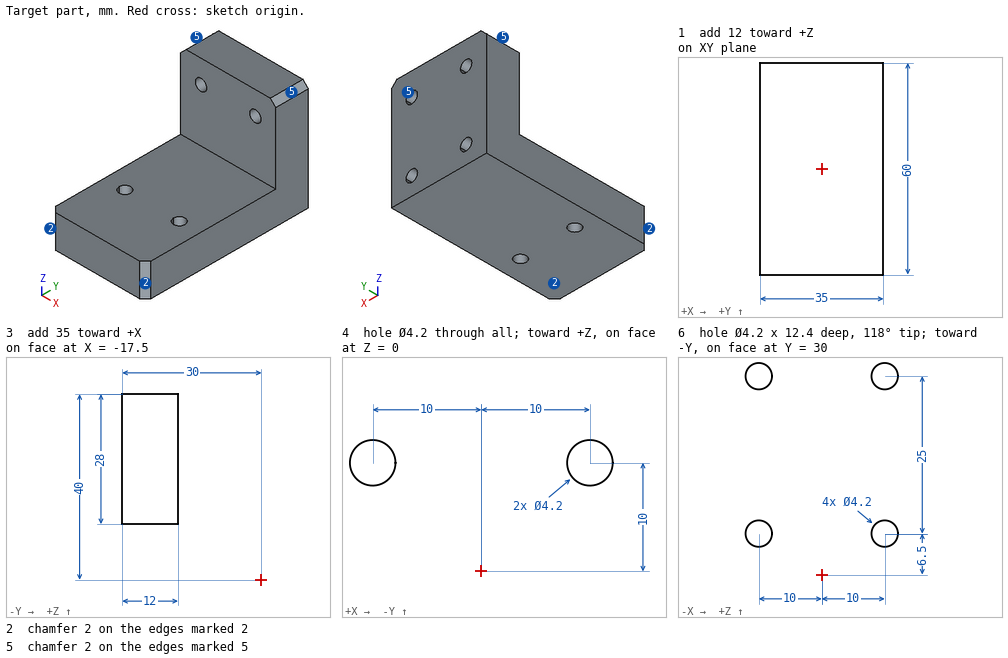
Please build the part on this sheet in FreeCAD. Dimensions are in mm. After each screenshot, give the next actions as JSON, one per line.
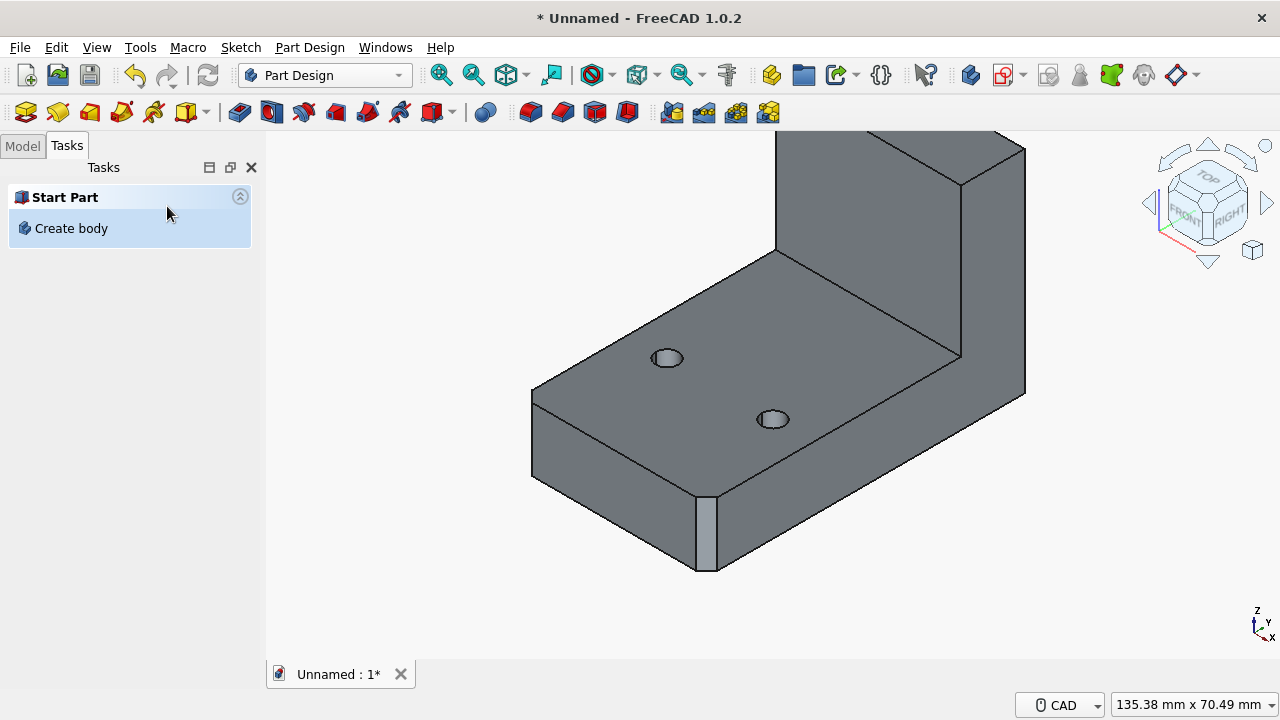
{"action": "left_click", "coordinate": [442, 76]}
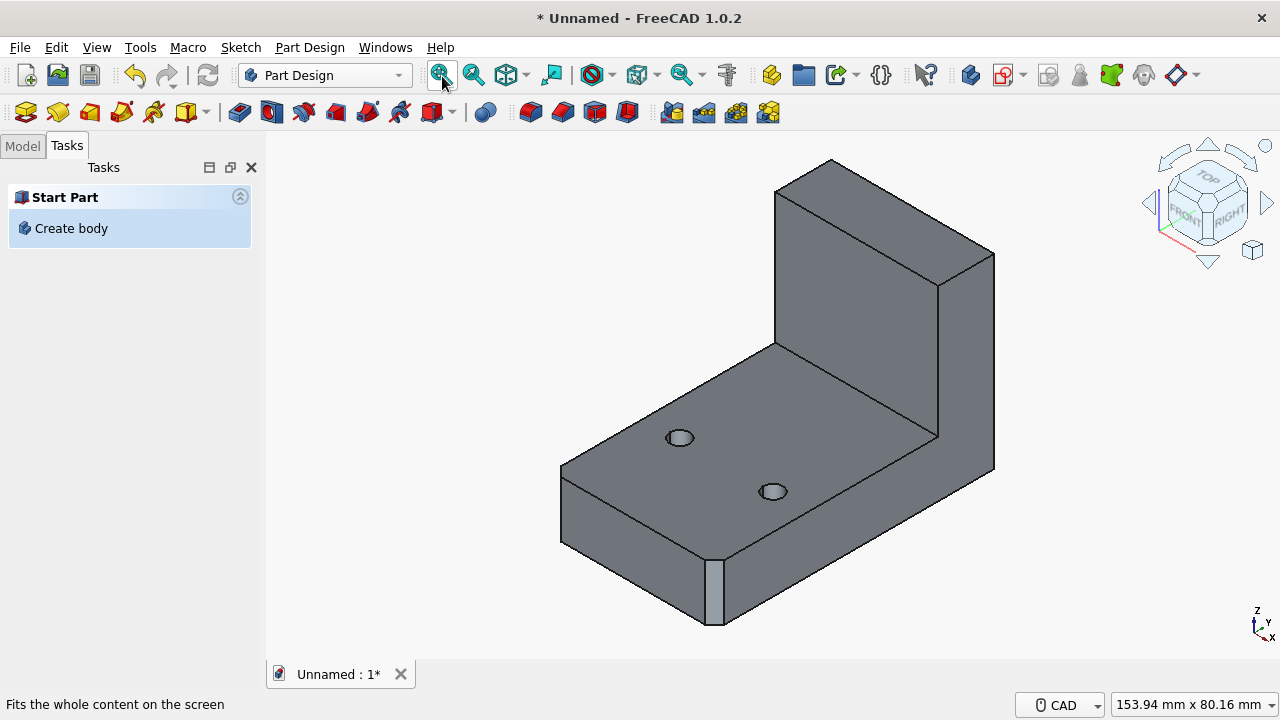
{"action": "left_click", "coordinate": [966, 269]}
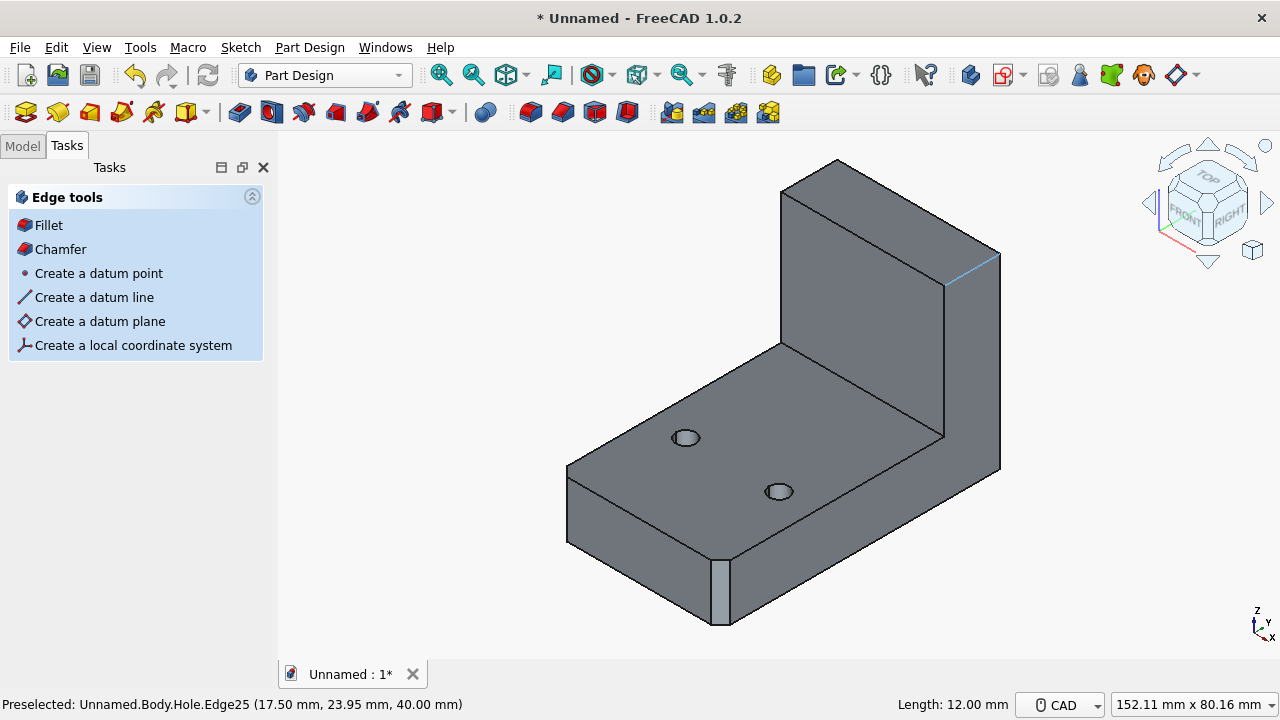
{"action": "key", "text": "2"}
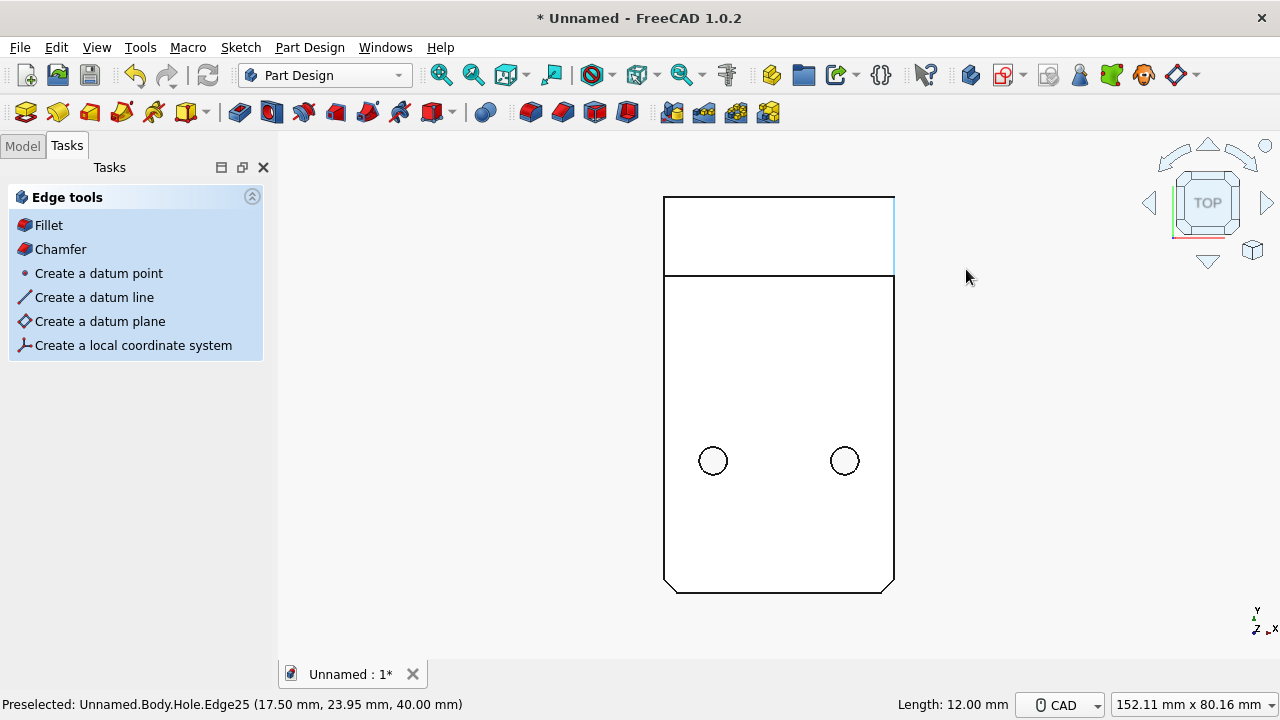
{"action": "left_click", "coordinate": [664, 236], "text": "ctrl"}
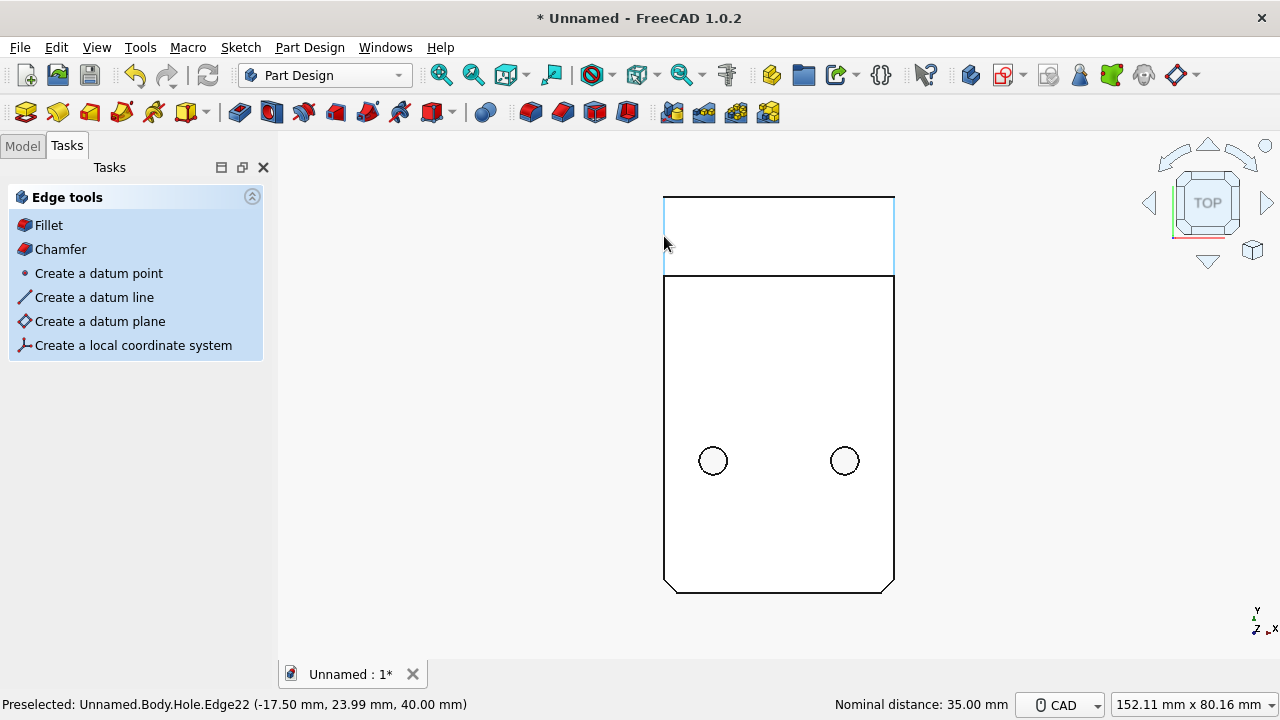
{"action": "left_click", "coordinate": [564, 112]}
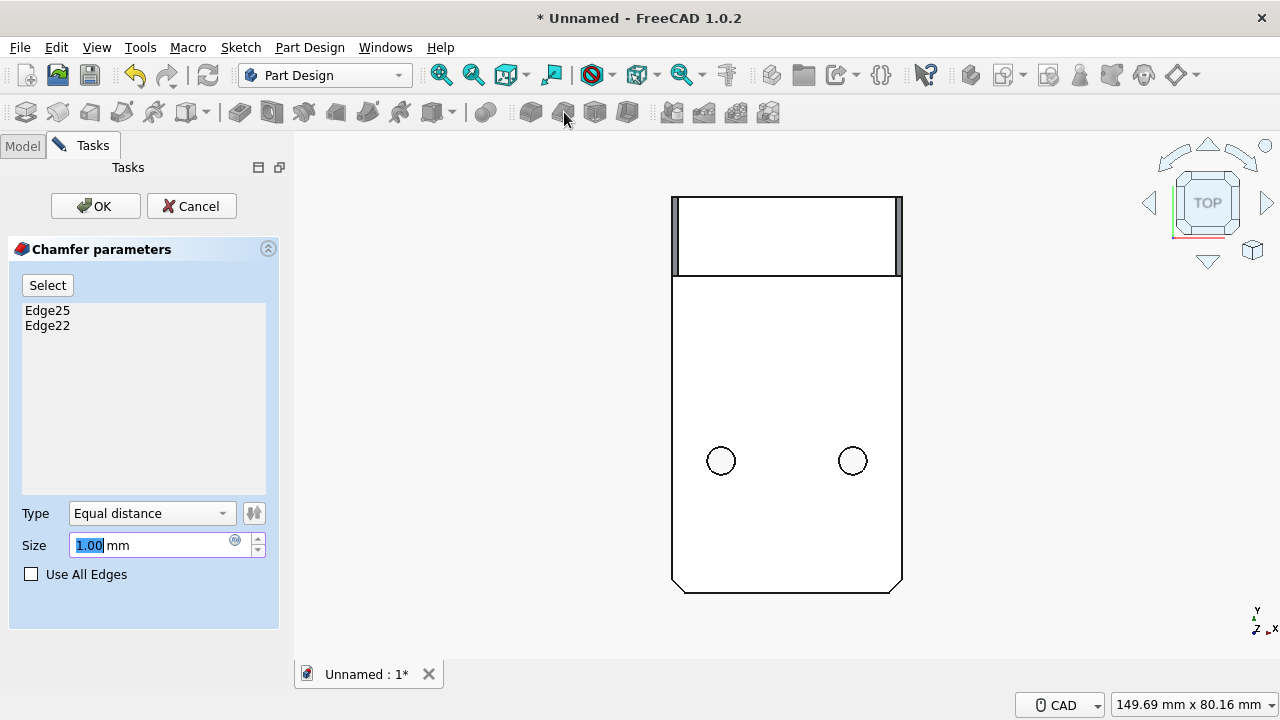
{"action": "type", "text": "2"}
{"action": "key", "text": "Tab"}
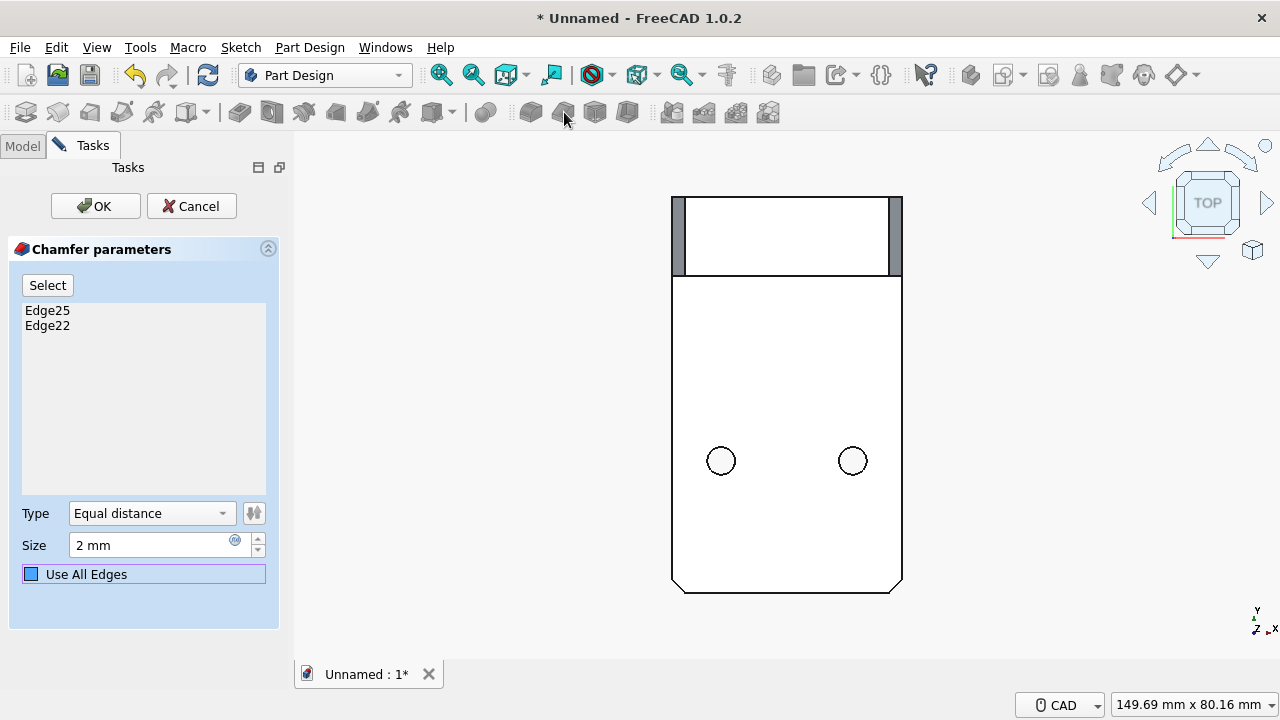
{"action": "left_click", "coordinate": [96, 206]}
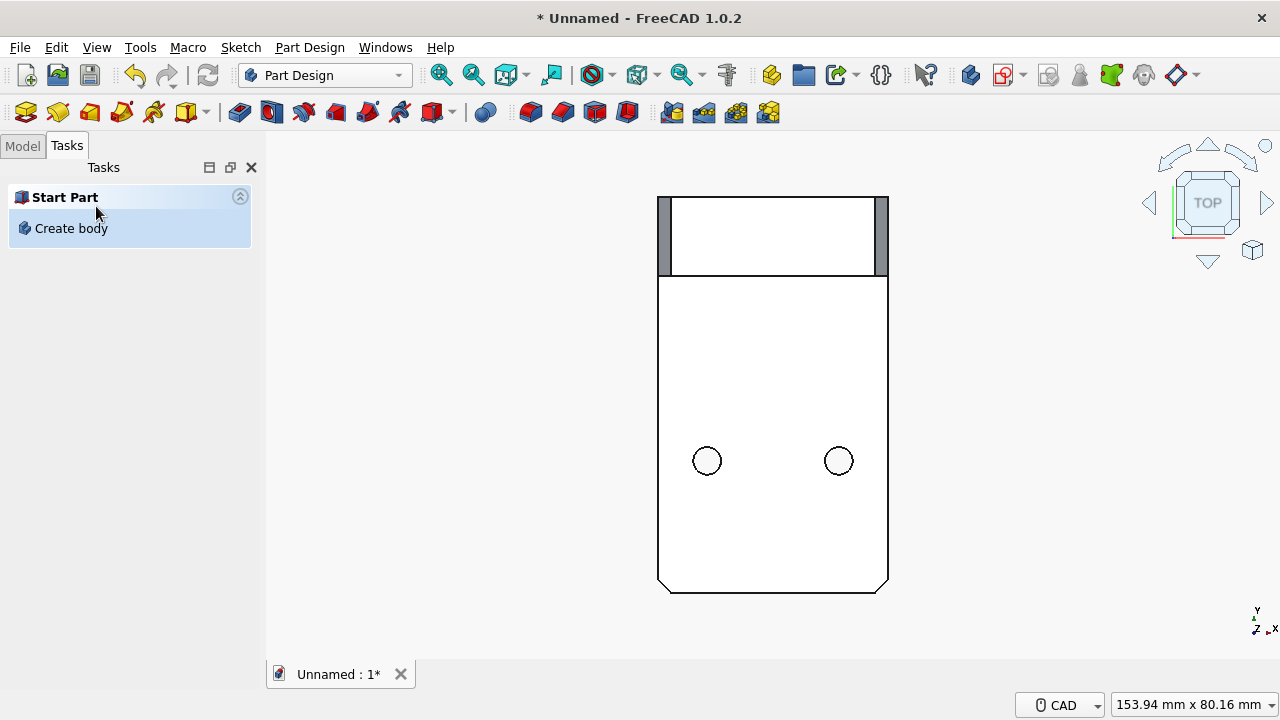
{"action": "key", "text": "4"}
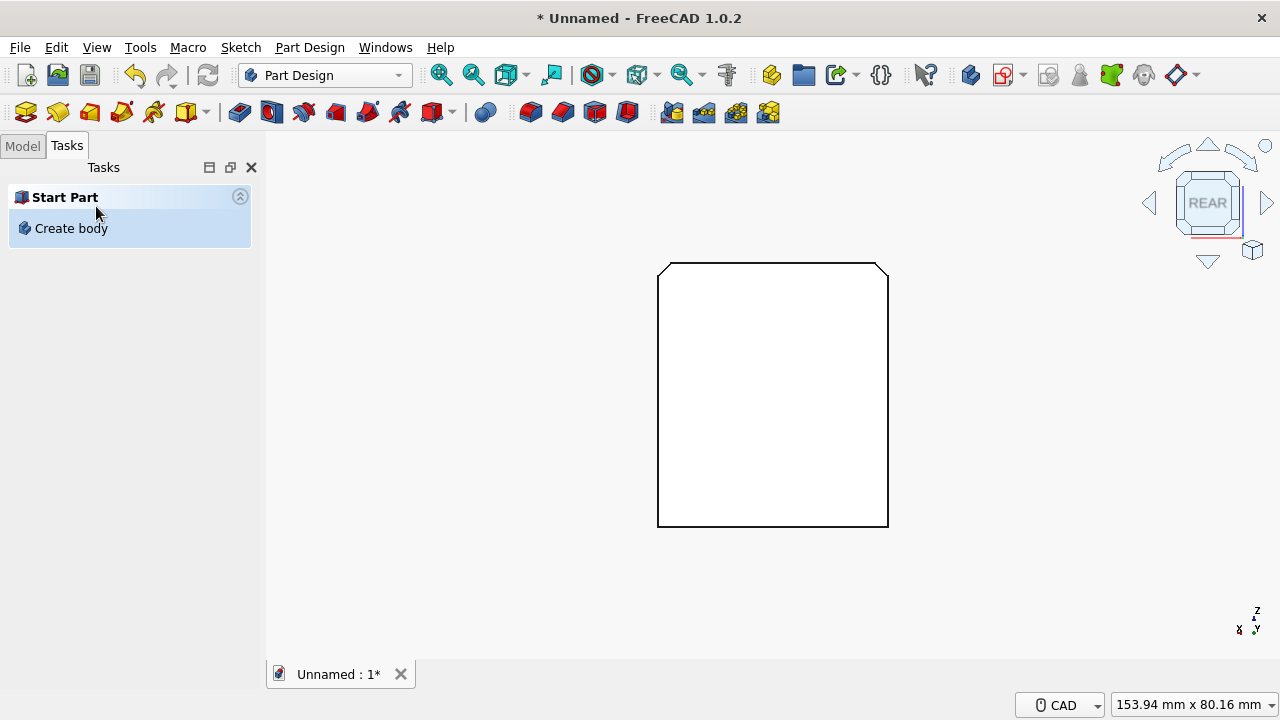
{"action": "left_click", "coordinate": [773, 394]}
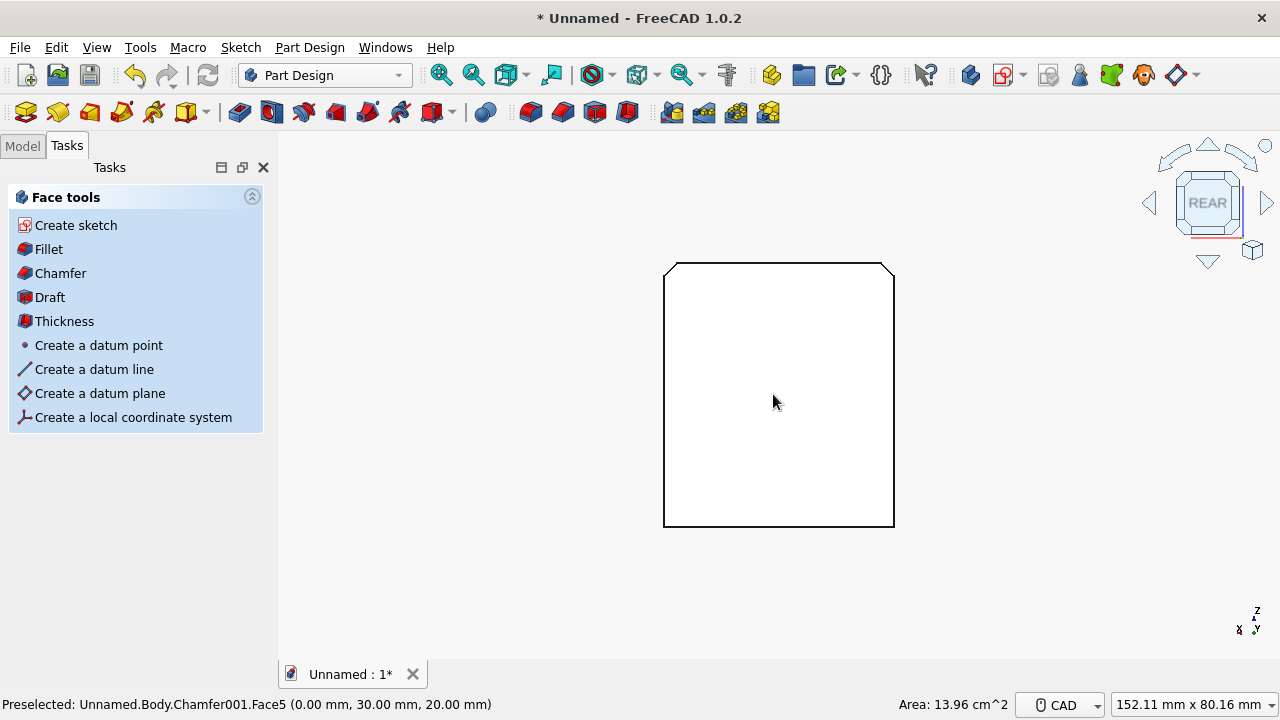
{"action": "left_click", "coordinate": [1004, 76]}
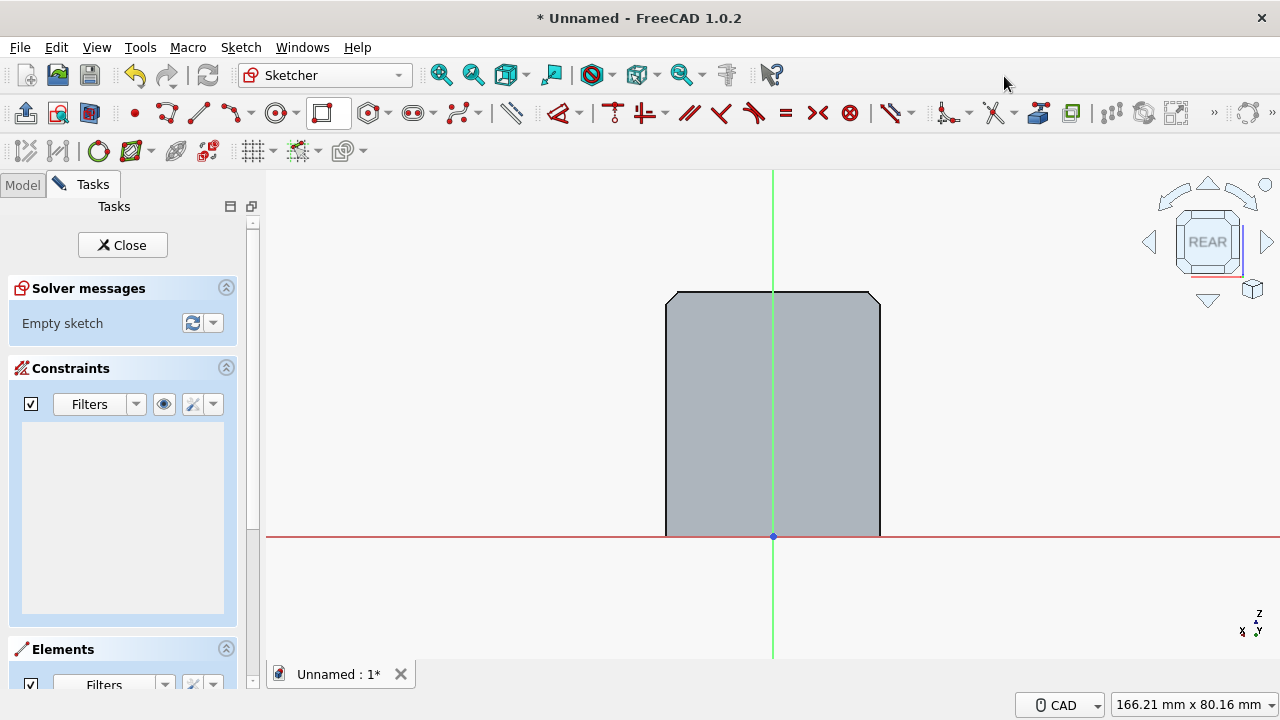
{"action": "scroll", "coordinate": [912, 474], "scroll_direction": "up", "scroll_amount": 2}